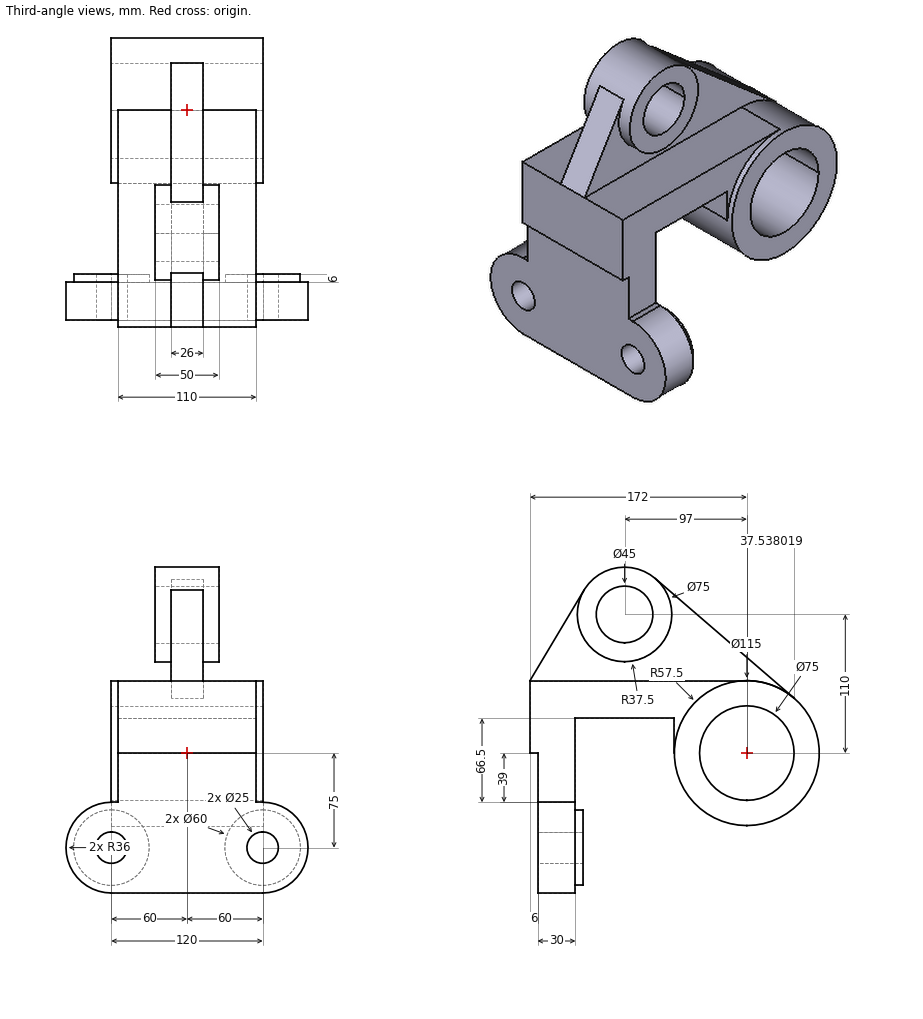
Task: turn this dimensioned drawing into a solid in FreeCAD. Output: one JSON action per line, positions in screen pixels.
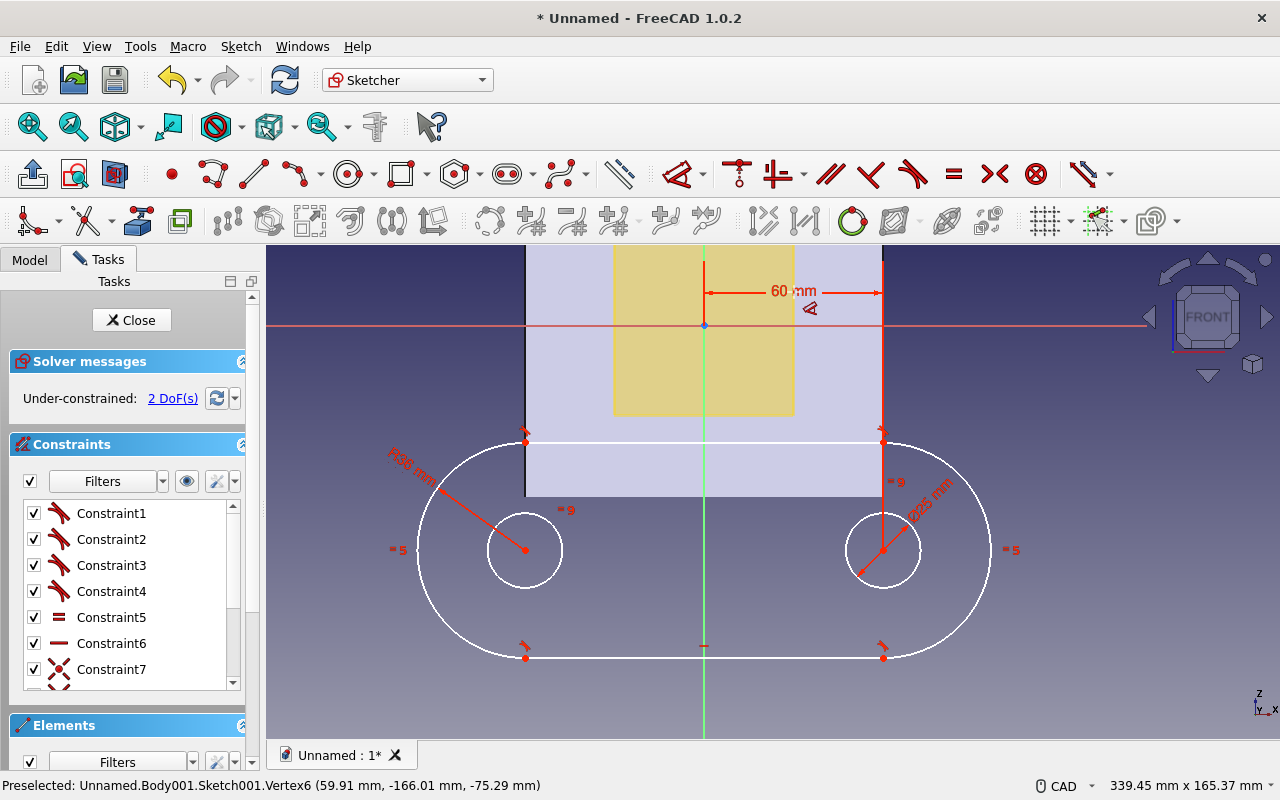
{"action": "left_click", "coordinate": [883, 551]}
{"action": "left_click", "coordinate": [917, 386]}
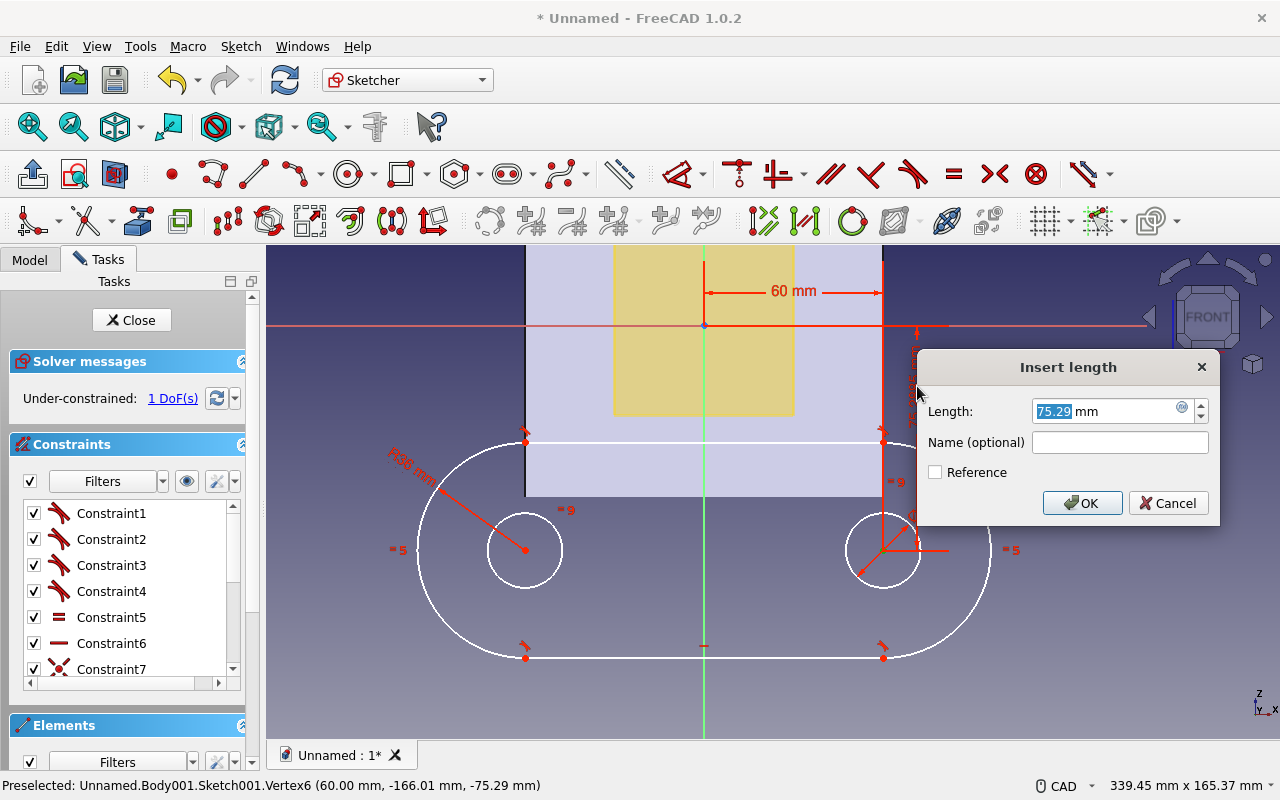
{"action": "type", "text": "75"}
{"action": "key", "text": "Return"}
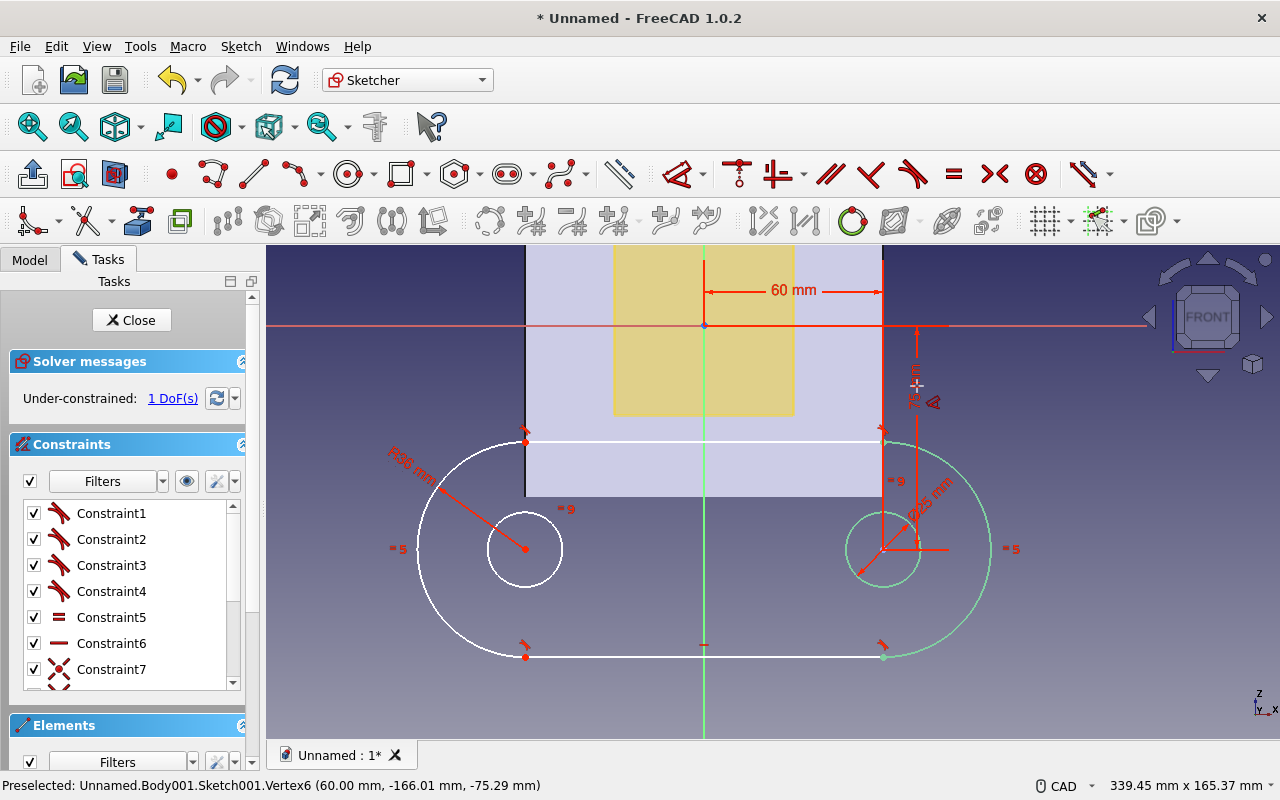
{"action": "left_click", "coordinate": [525, 550]}
{"action": "left_click", "coordinate": [615, 292]}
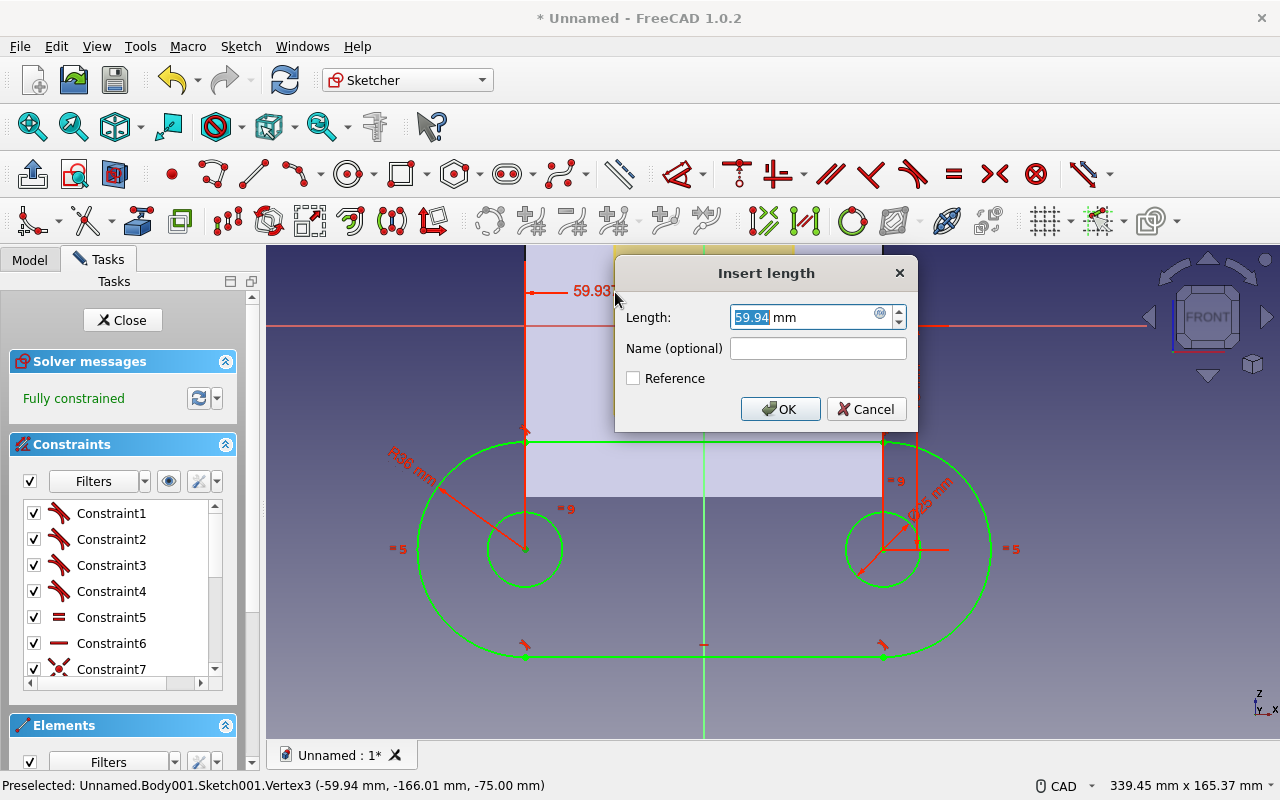
{"action": "type", "text": "60"}
{"action": "key", "text": "Return"}
{"action": "key", "text": "Escape"}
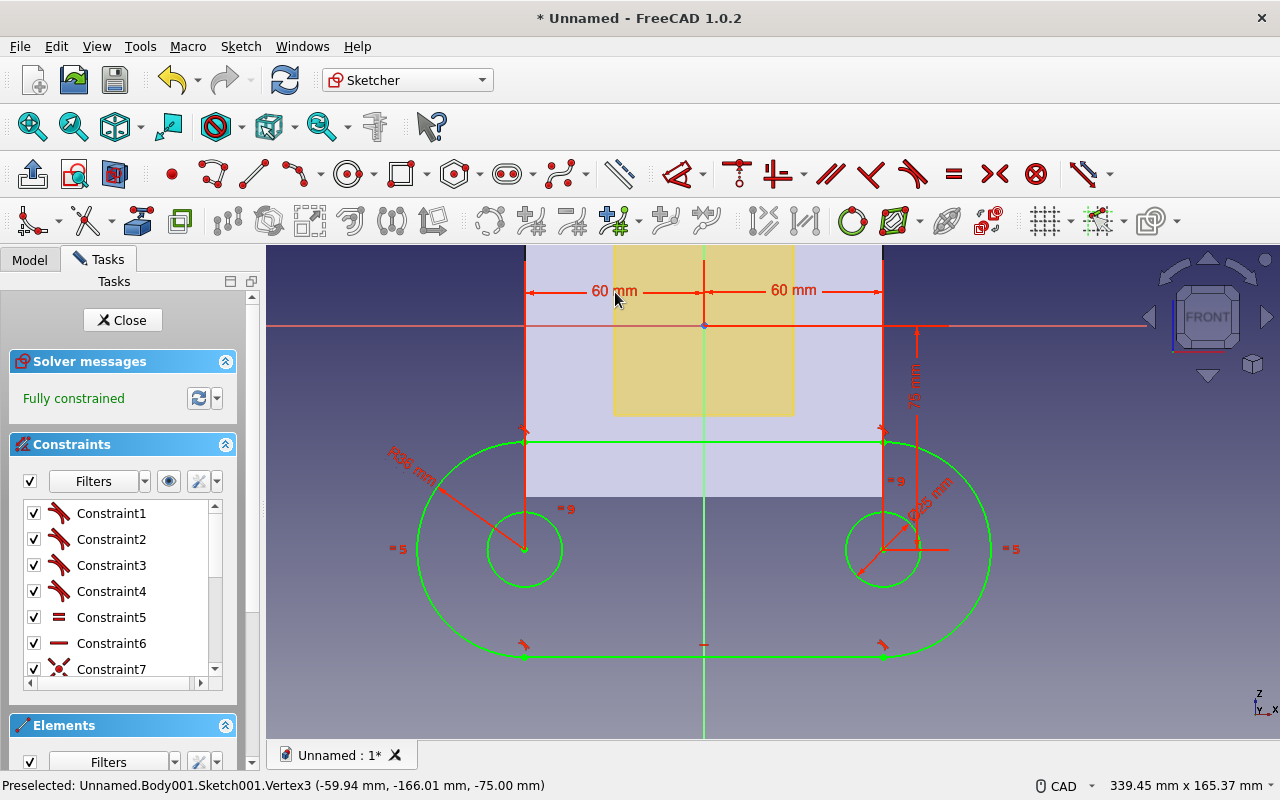
{"action": "left_click", "coordinate": [123, 320]}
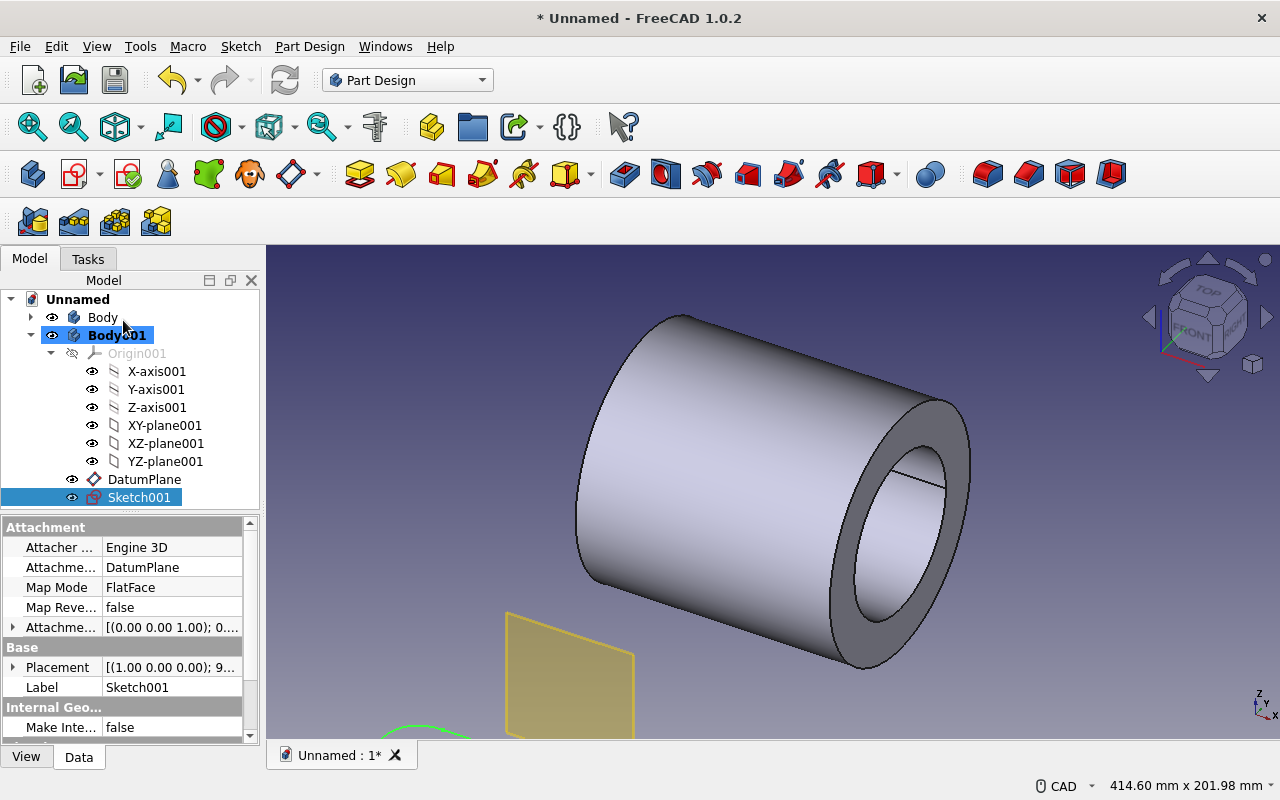
{"action": "left_click", "coordinate": [360, 174]}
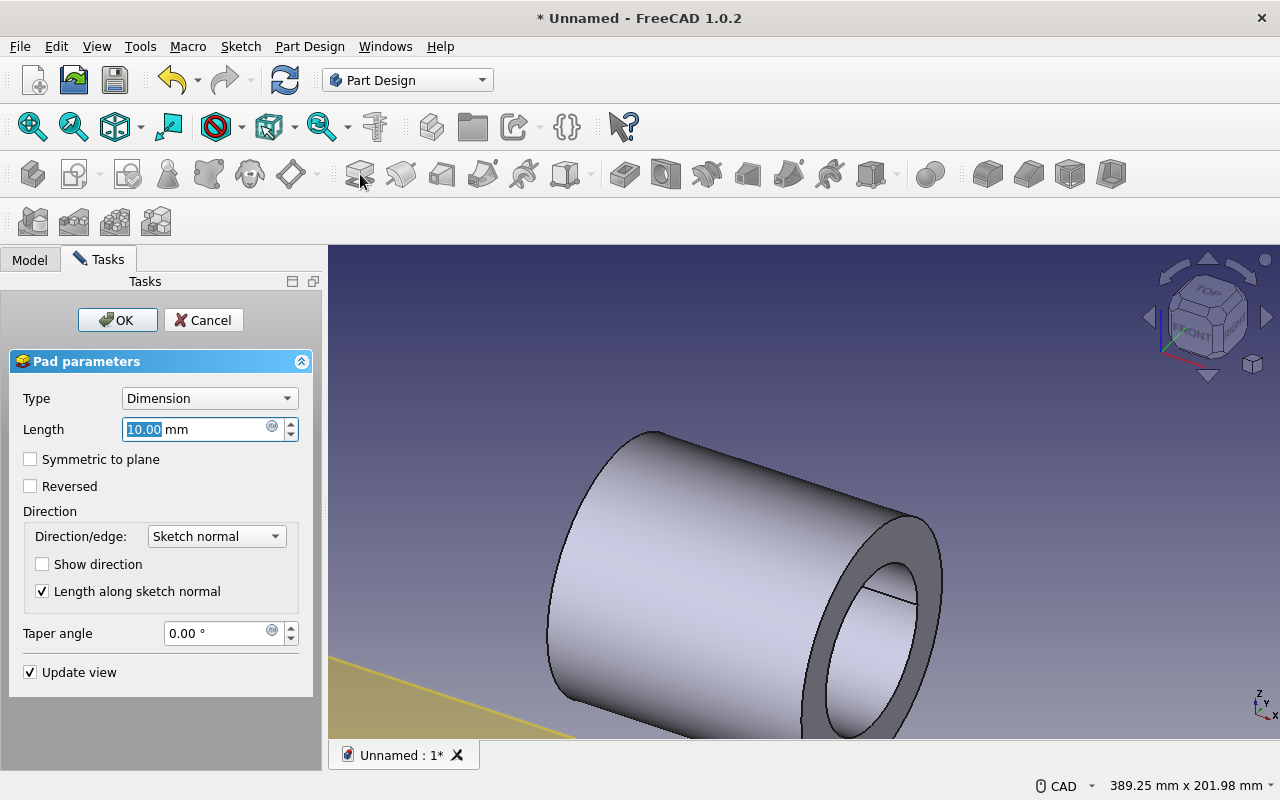
{"action": "type", "text": "30"}
{"action": "key", "text": "Tab"}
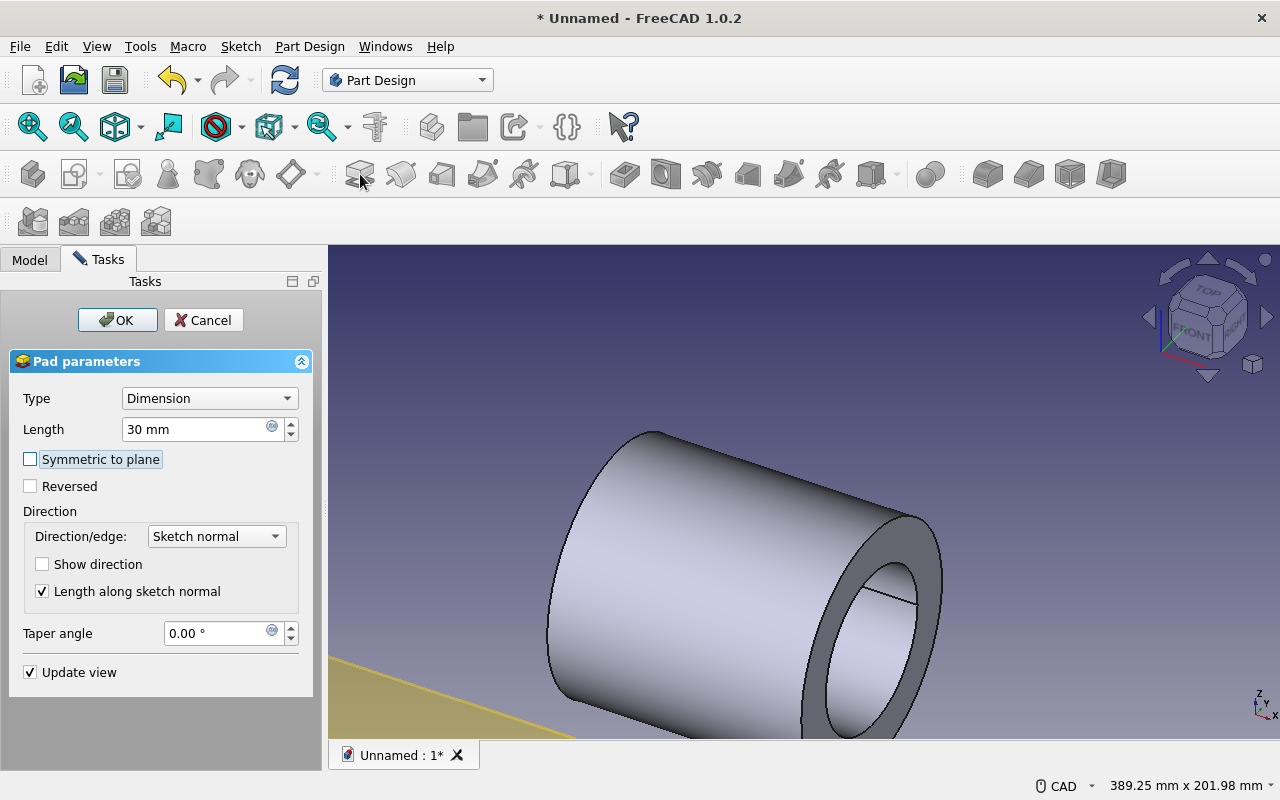
{"action": "left_click", "coordinate": [31, 486]}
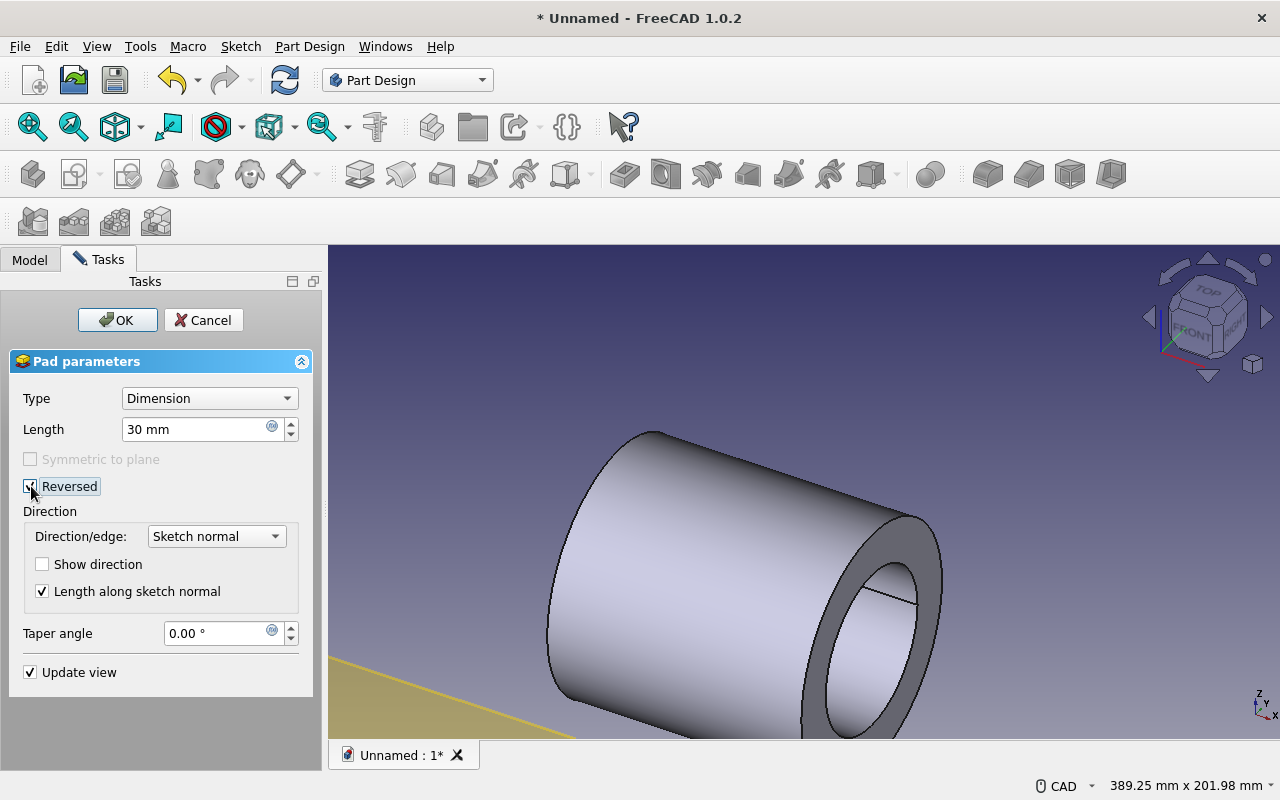
{"action": "left_click", "coordinate": [118, 320]}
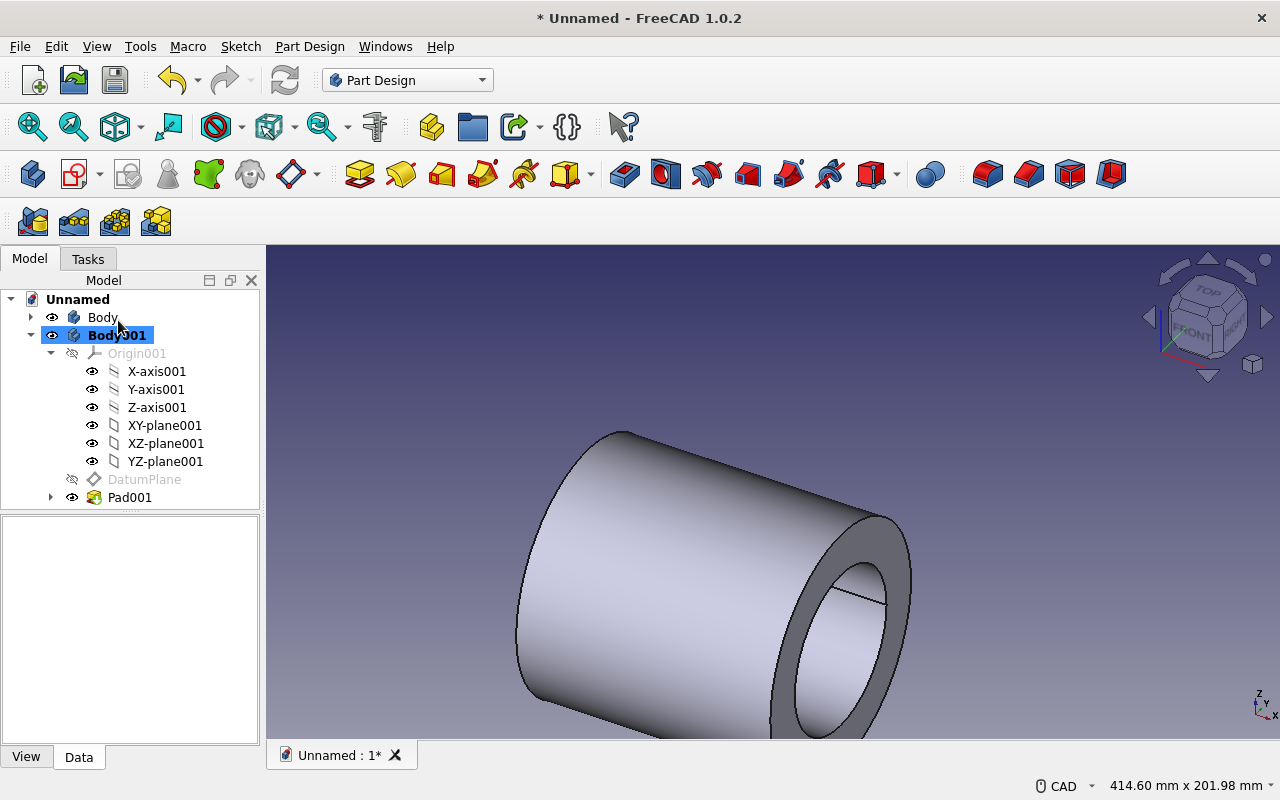
{"action": "key", "text": "v f"}